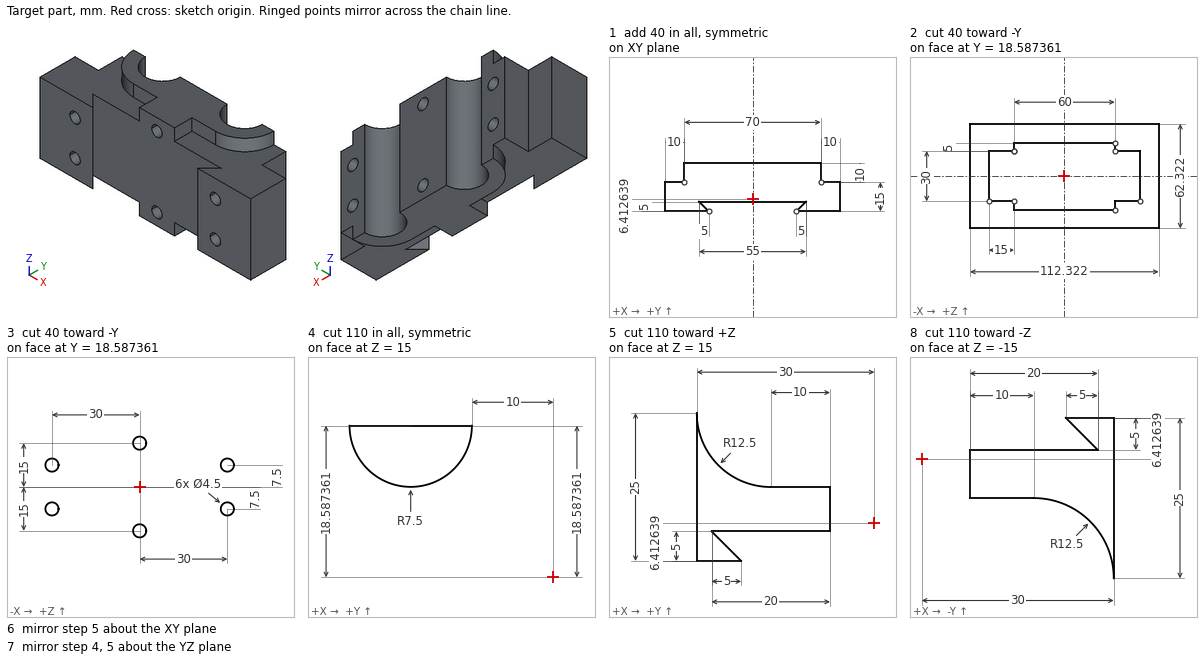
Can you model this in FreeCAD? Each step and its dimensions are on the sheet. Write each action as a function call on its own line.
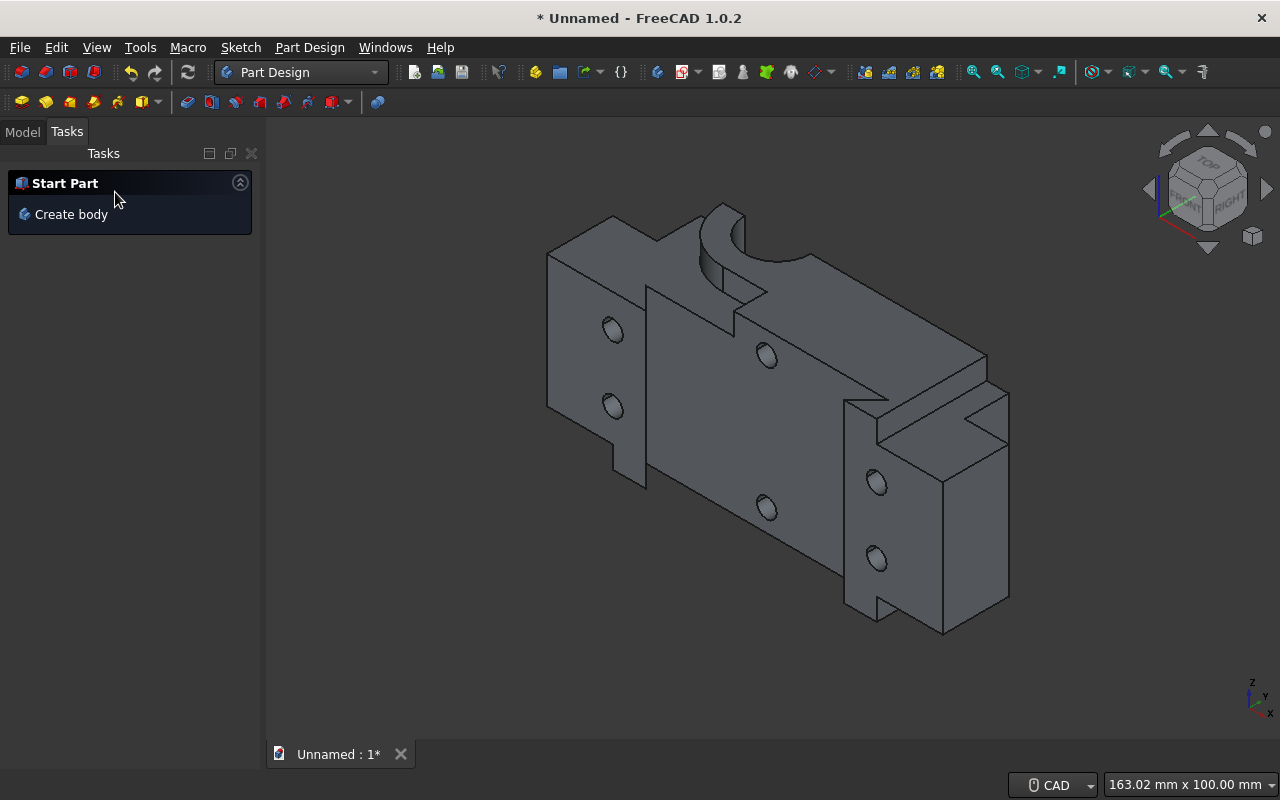
click(23, 131)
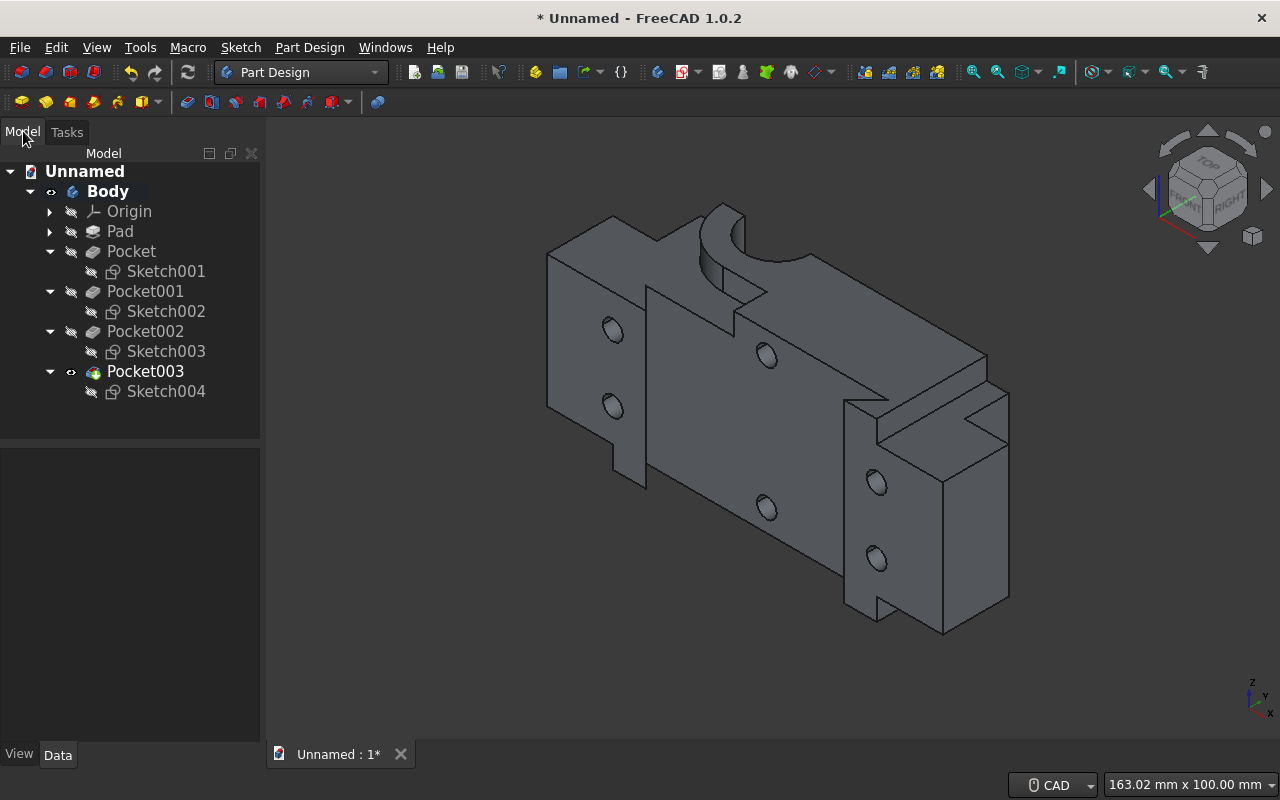
click(116, 372)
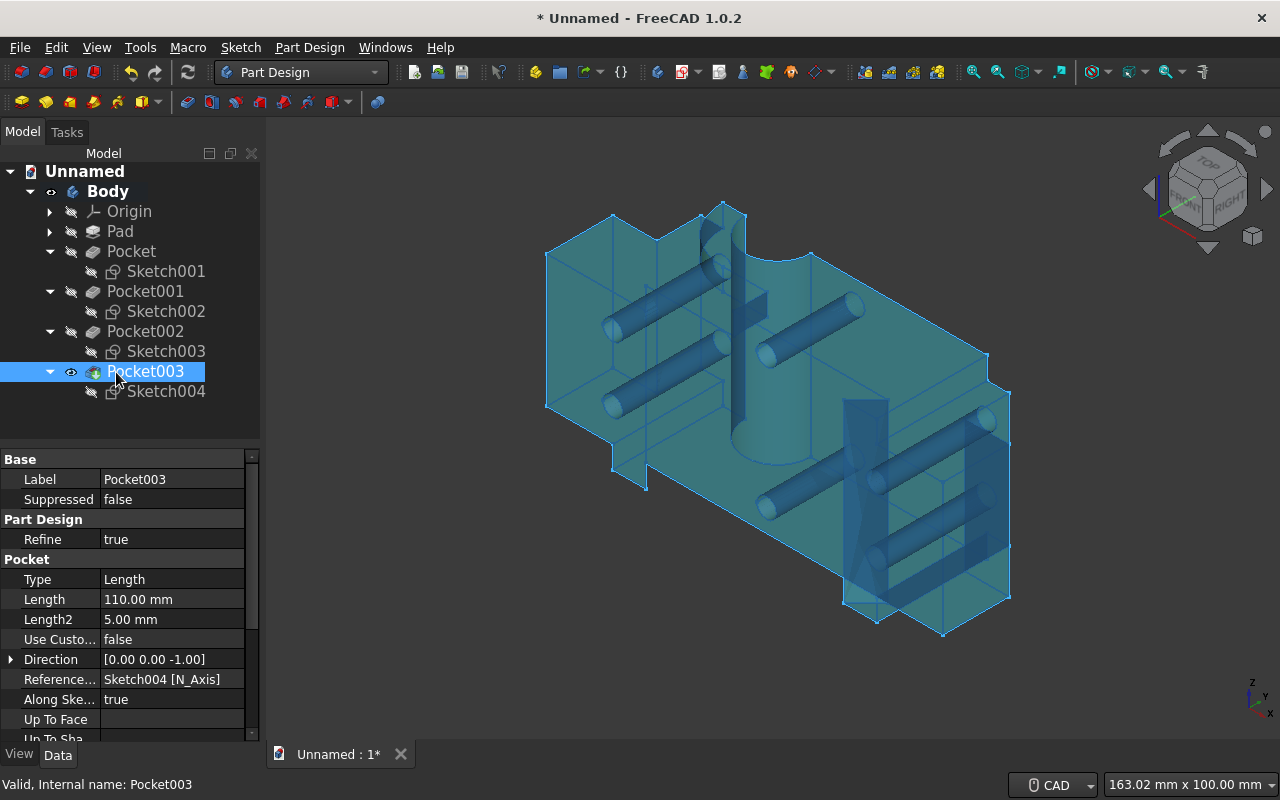
click(866, 72)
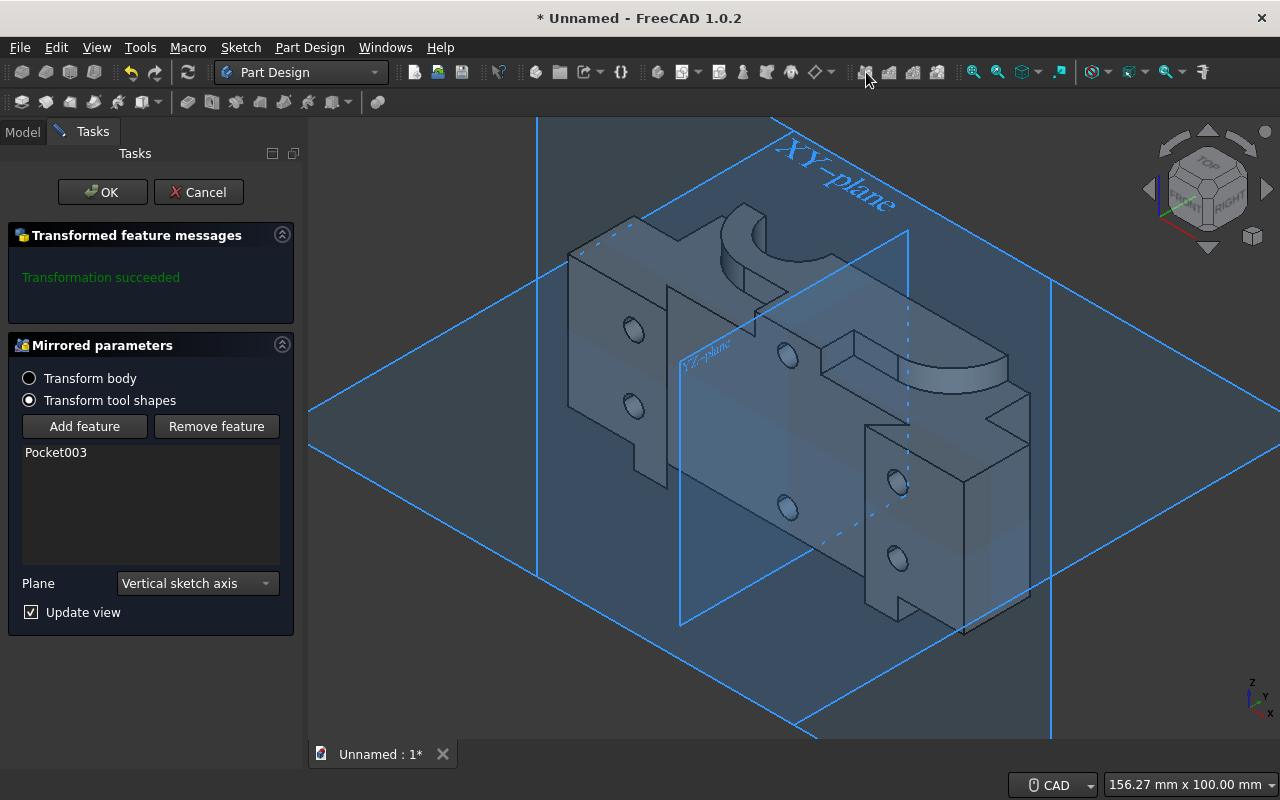
click(198, 584)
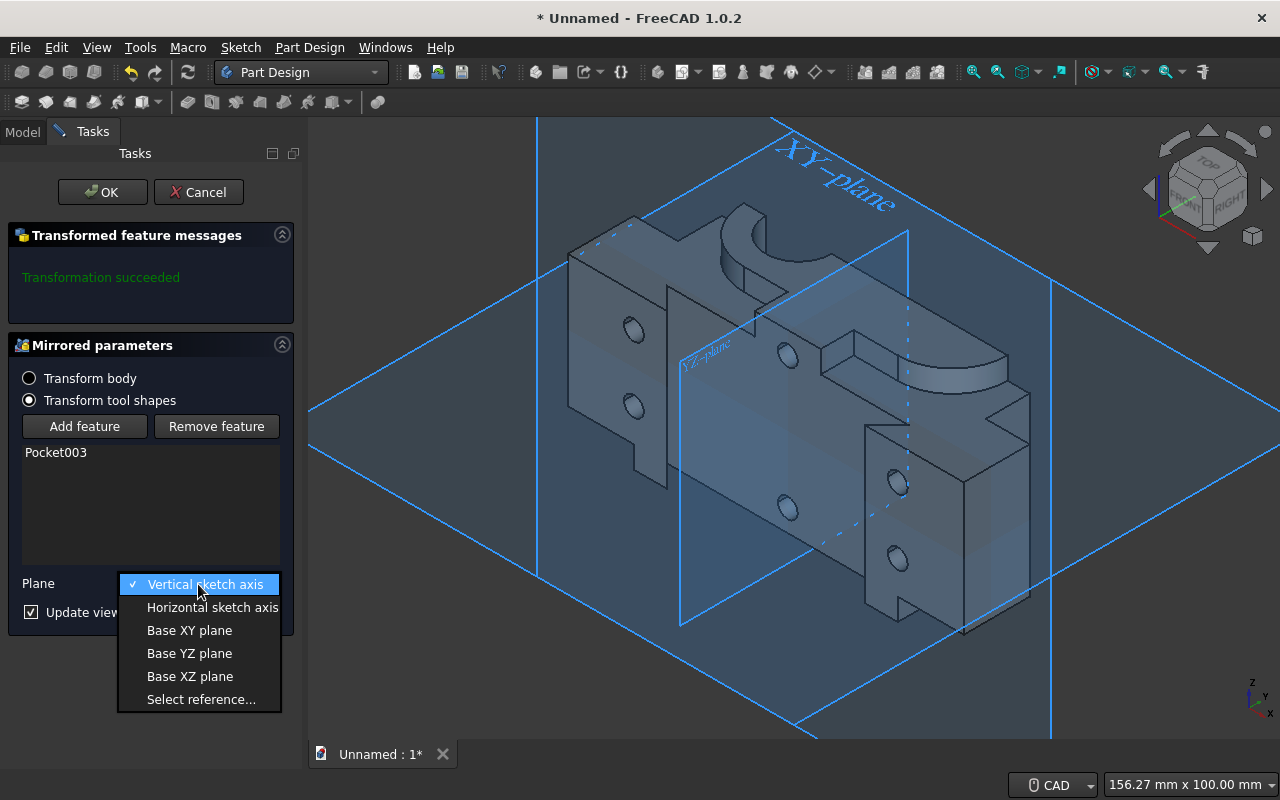
click(198, 630)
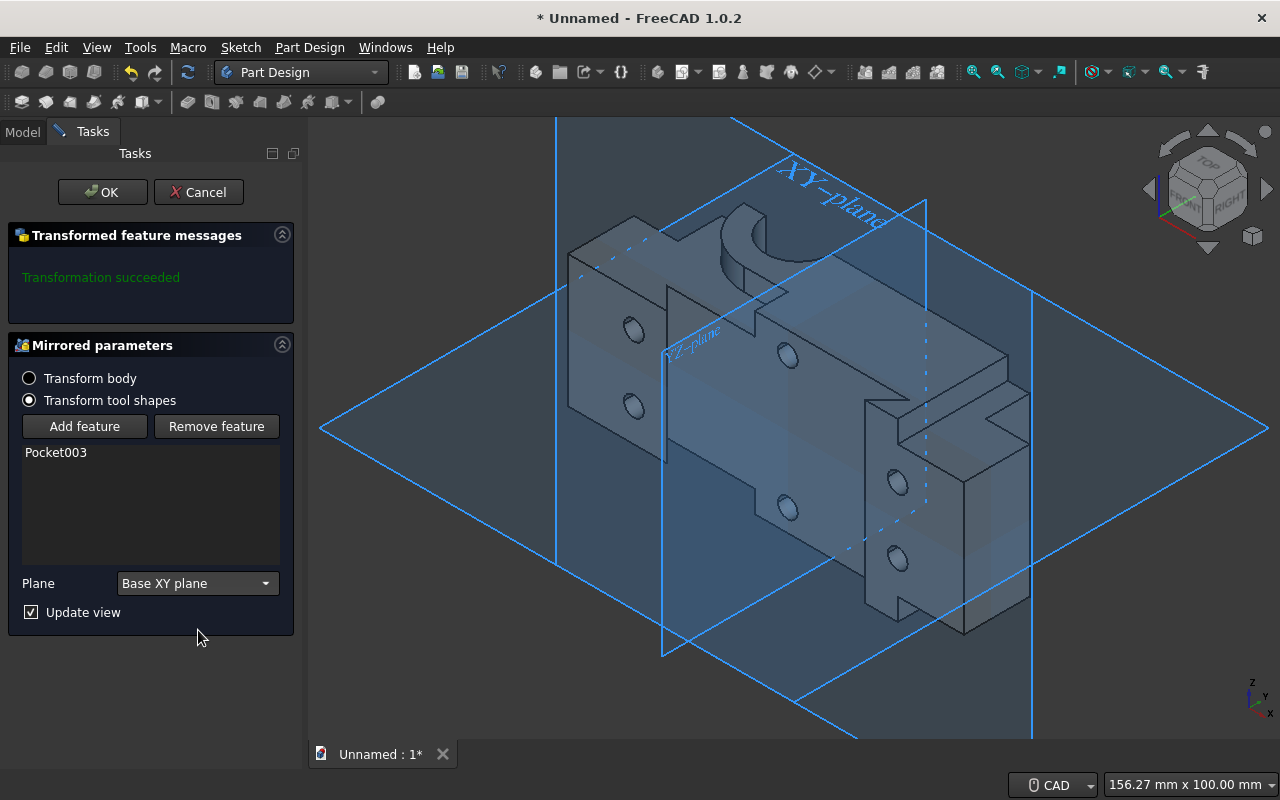
click(103, 192)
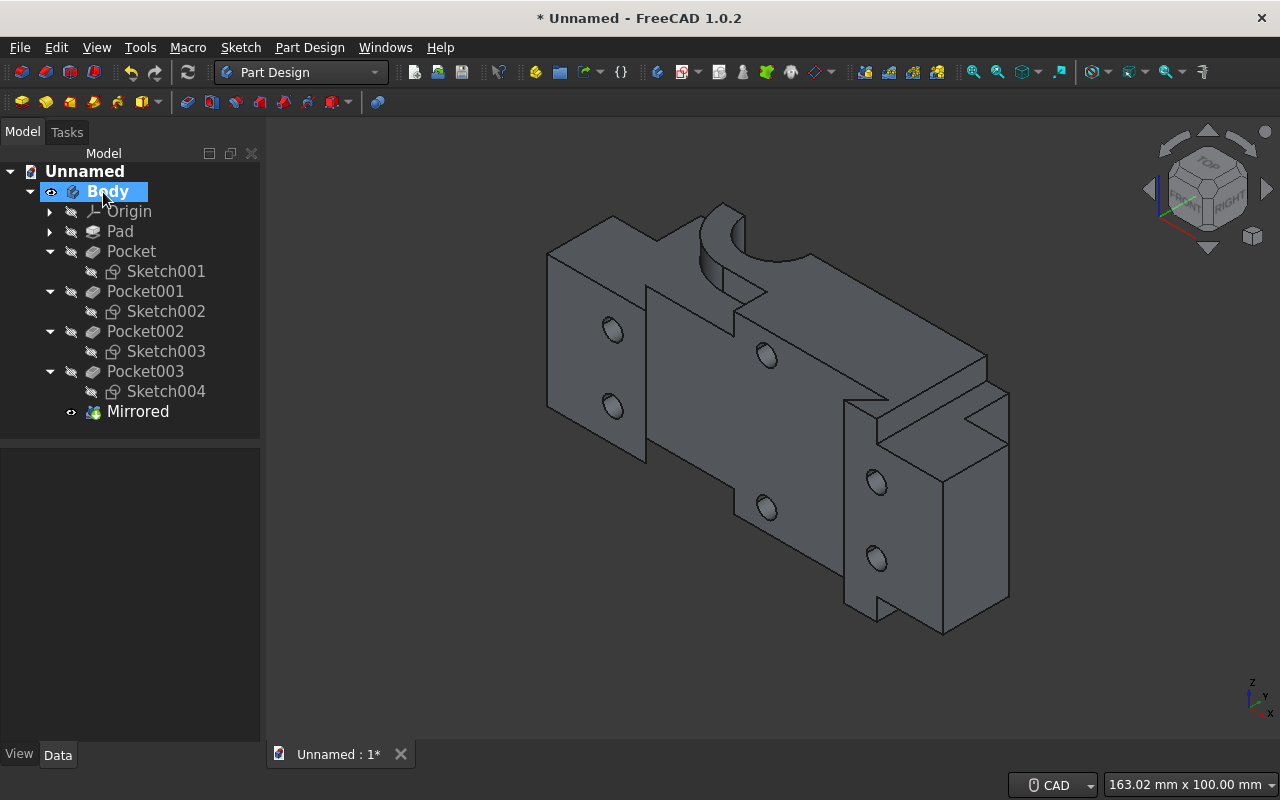
click(116, 332)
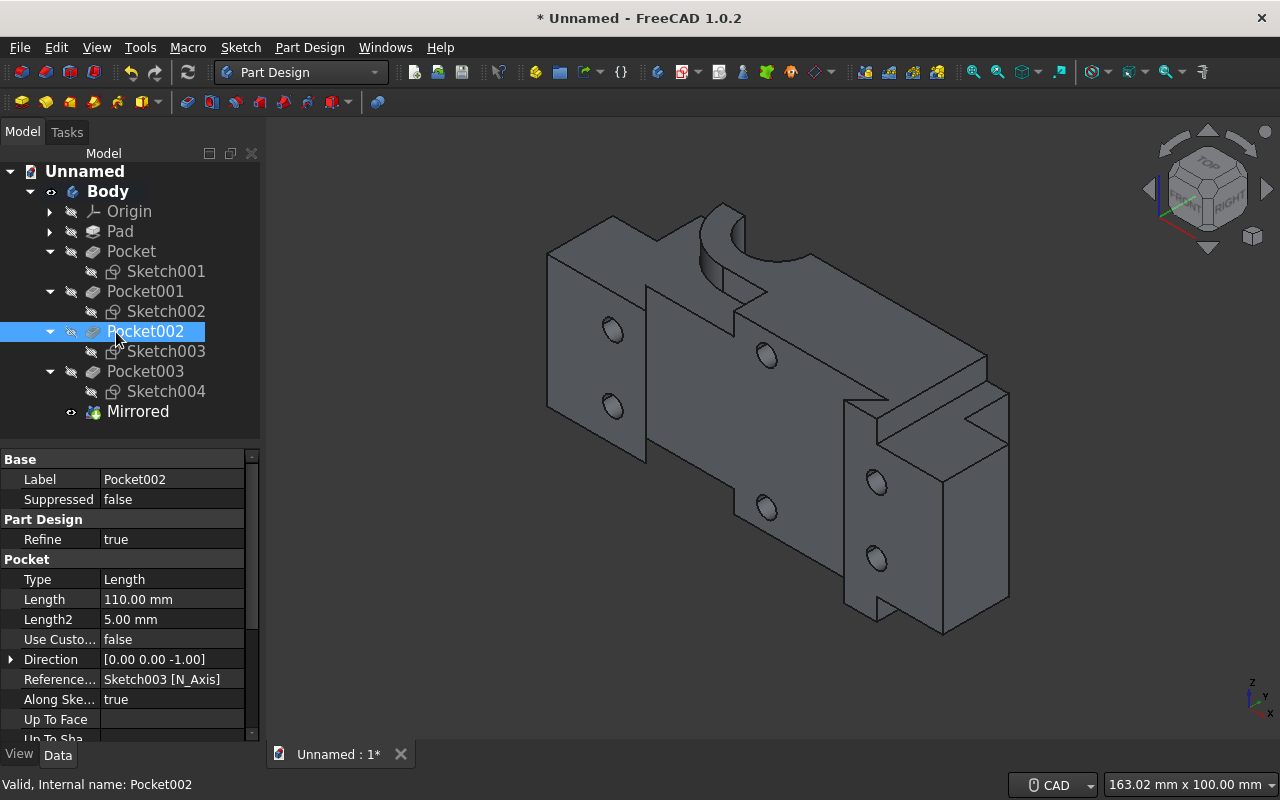
click(116, 372, ctrl)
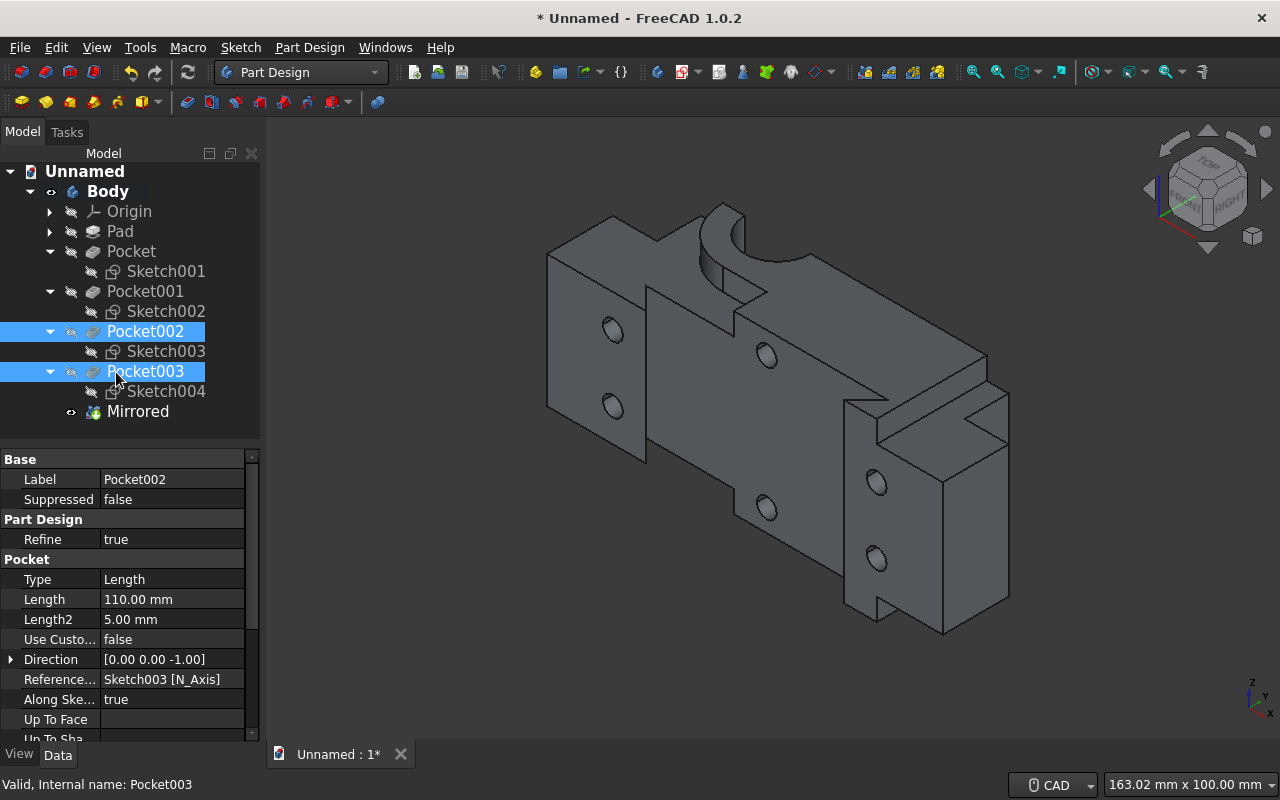
click(866, 72)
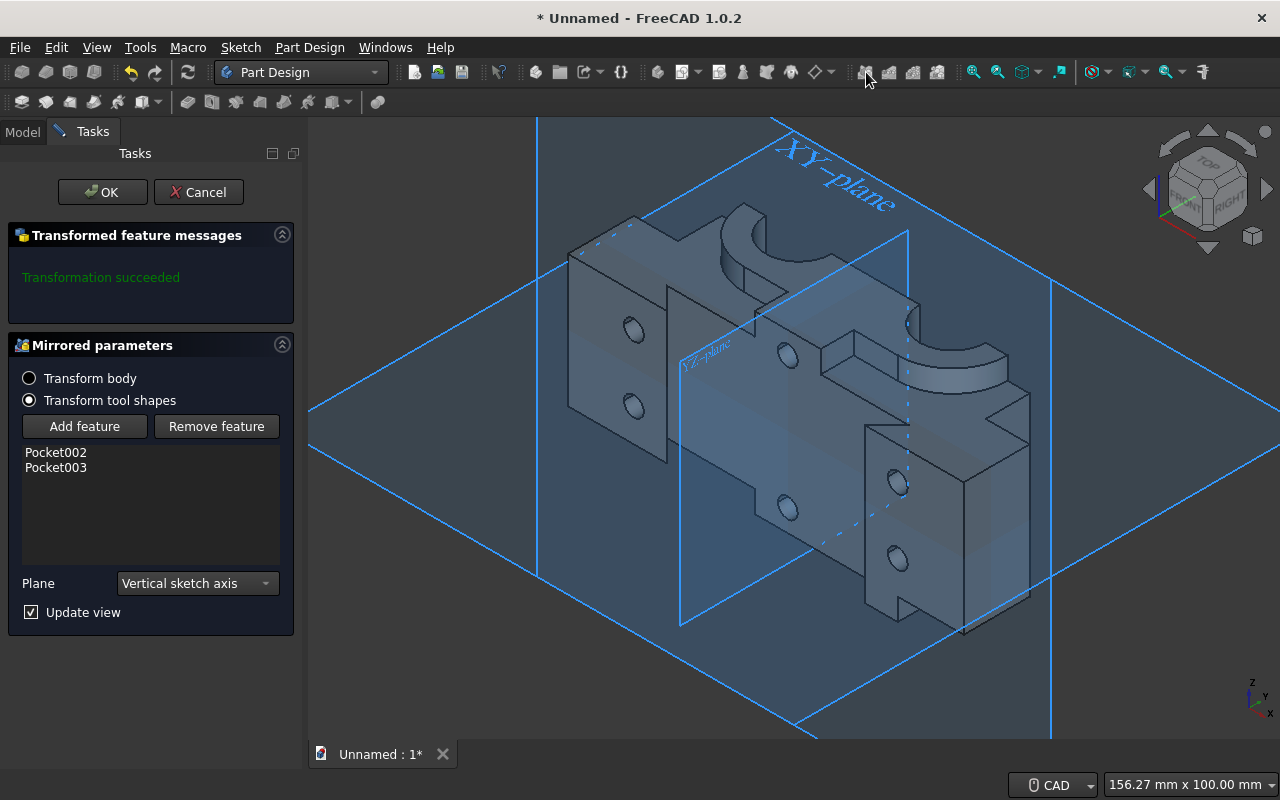
click(198, 584)